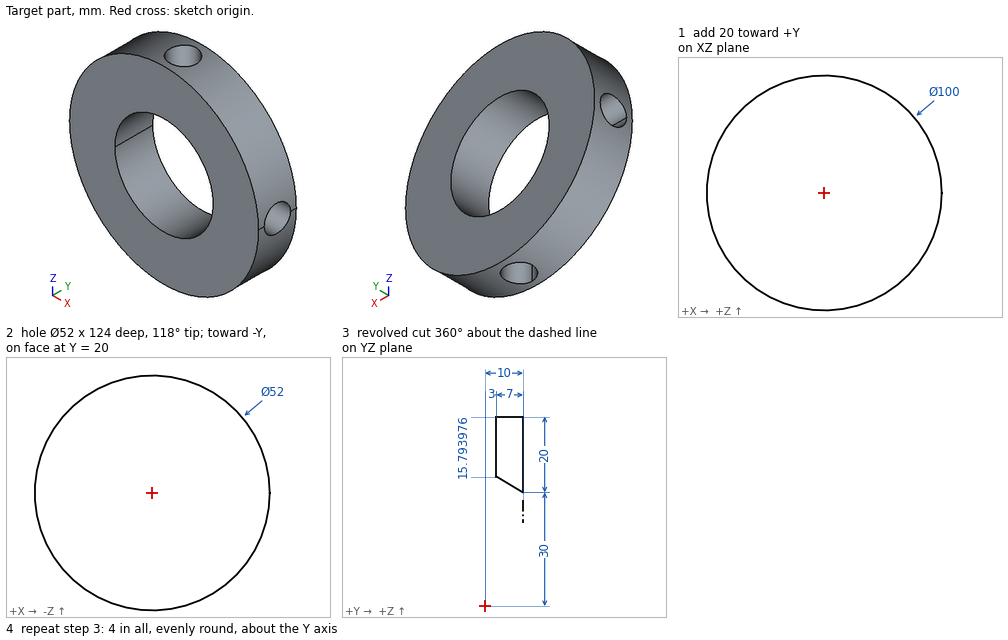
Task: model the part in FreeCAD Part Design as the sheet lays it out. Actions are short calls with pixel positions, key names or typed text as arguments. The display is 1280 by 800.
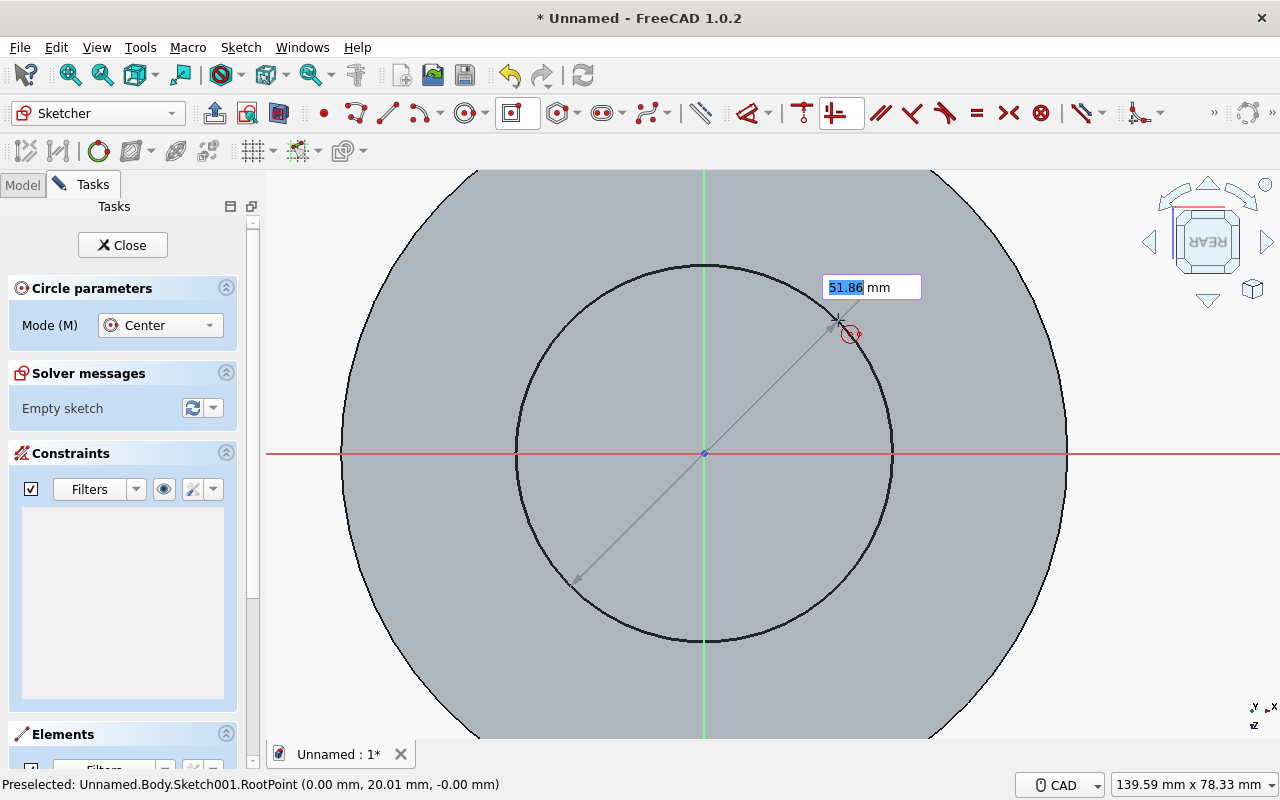
text(52)
key(Return)
key(Escape)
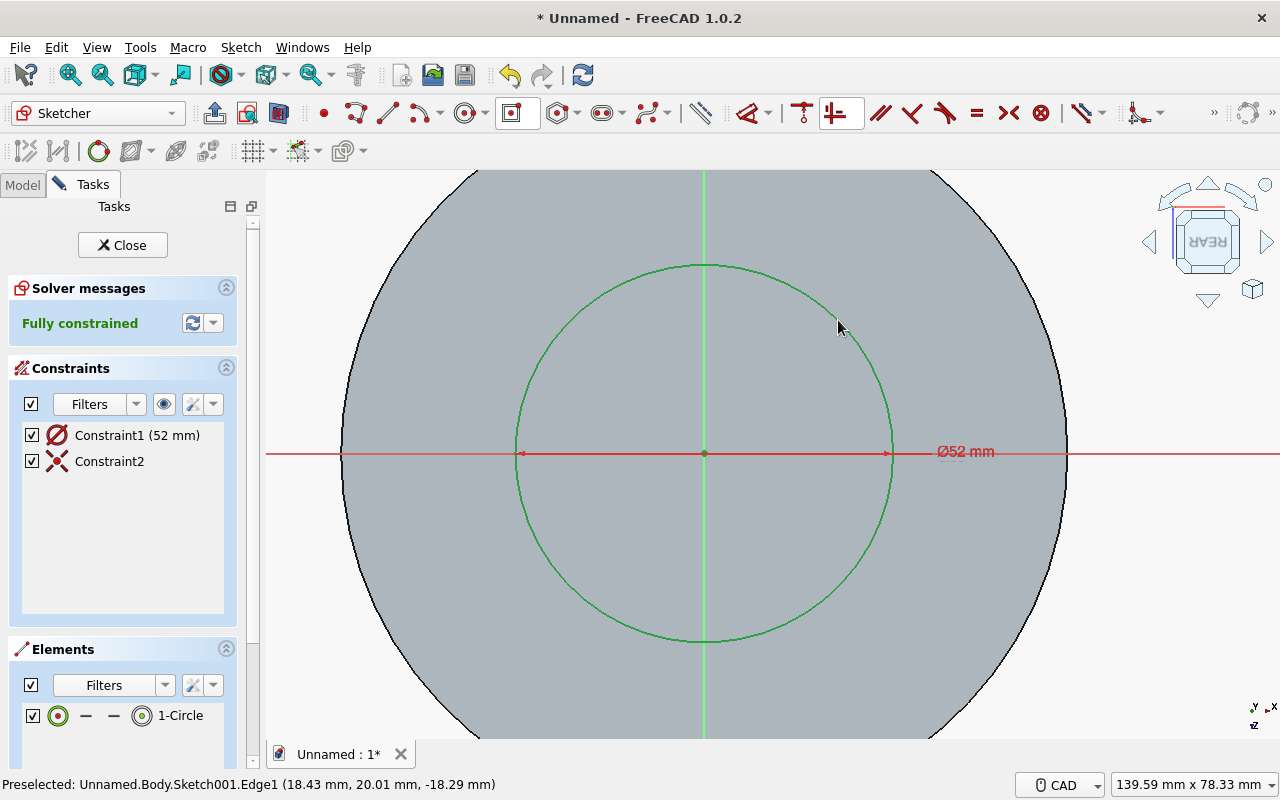
click(123, 245)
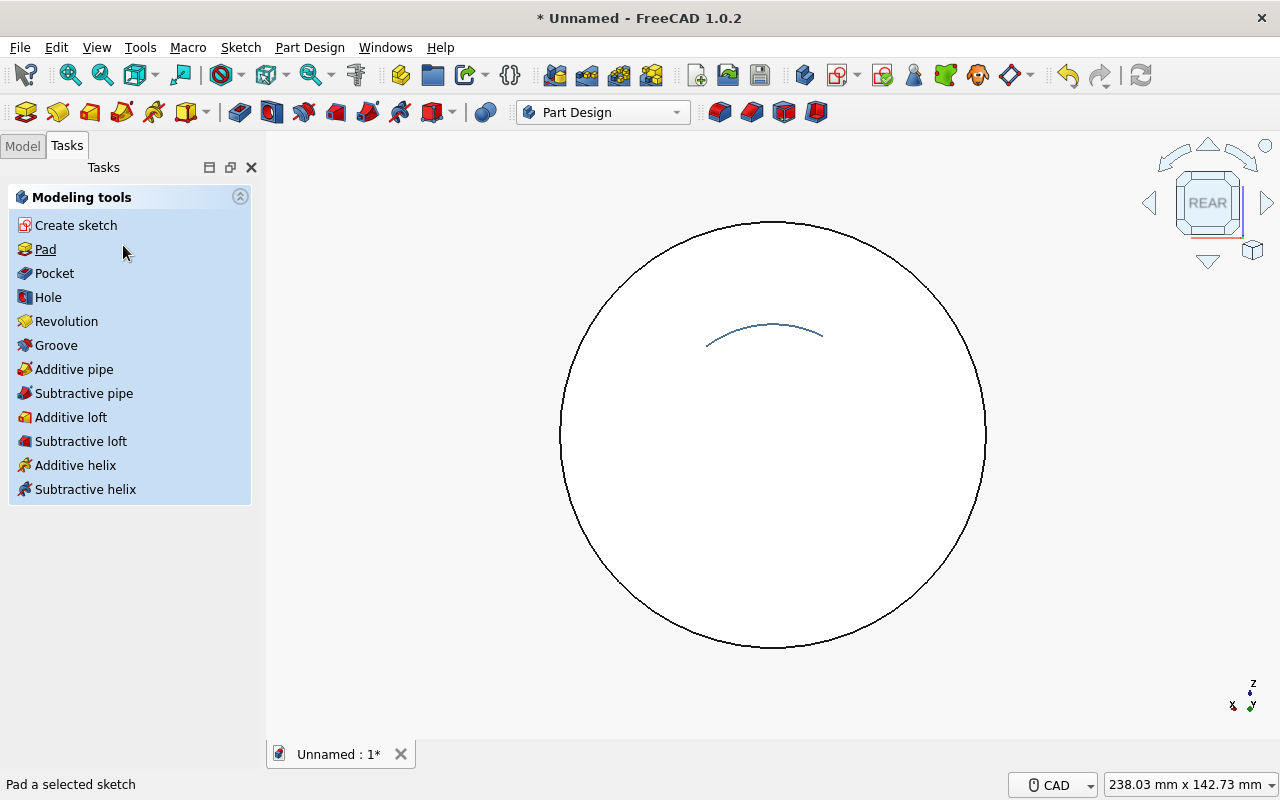
click(272, 112)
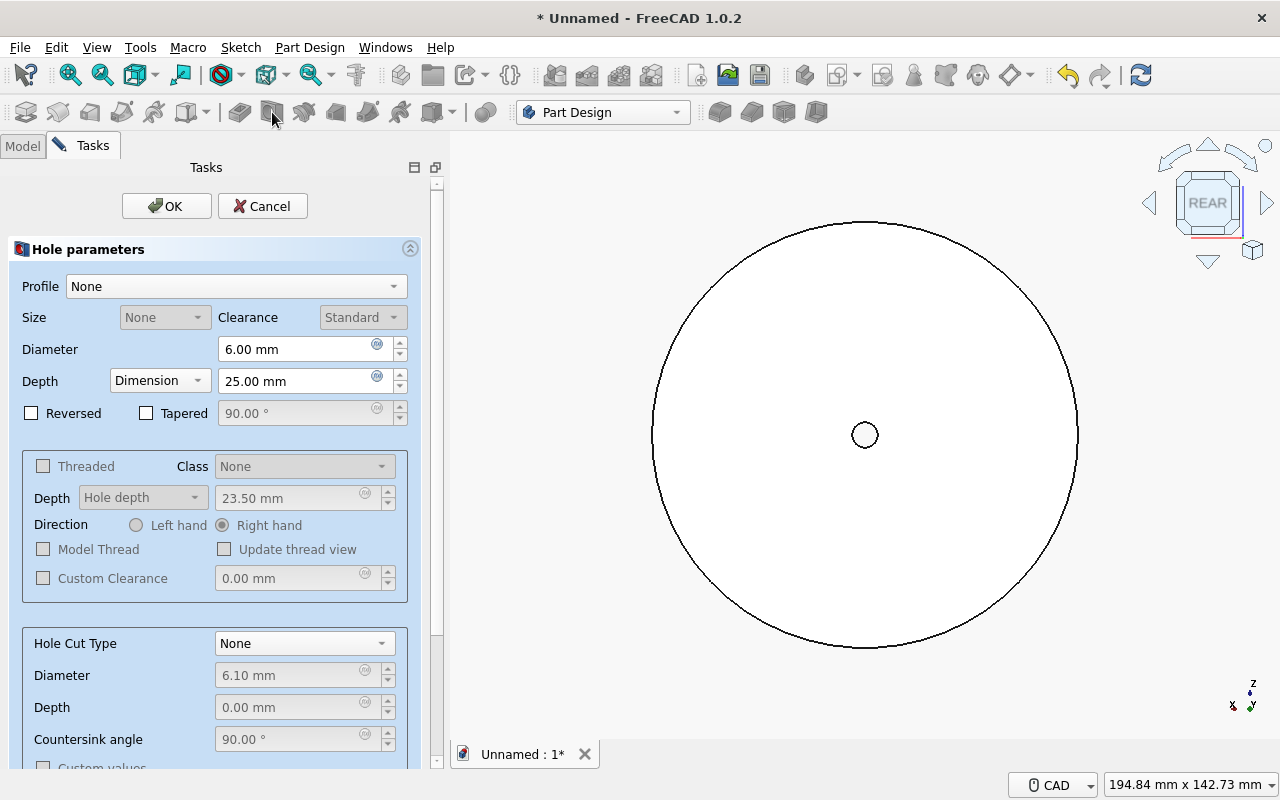
triple_click(305, 349)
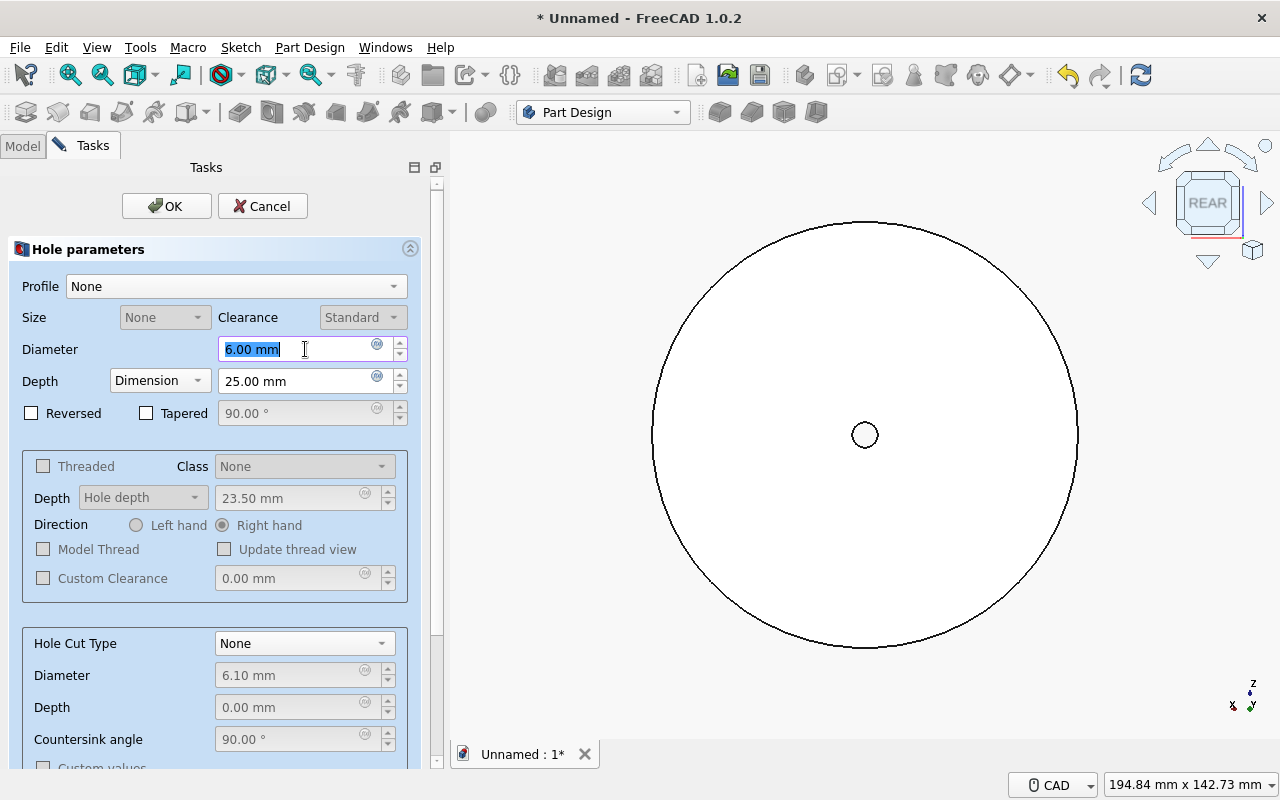
text(52)
key(Tab)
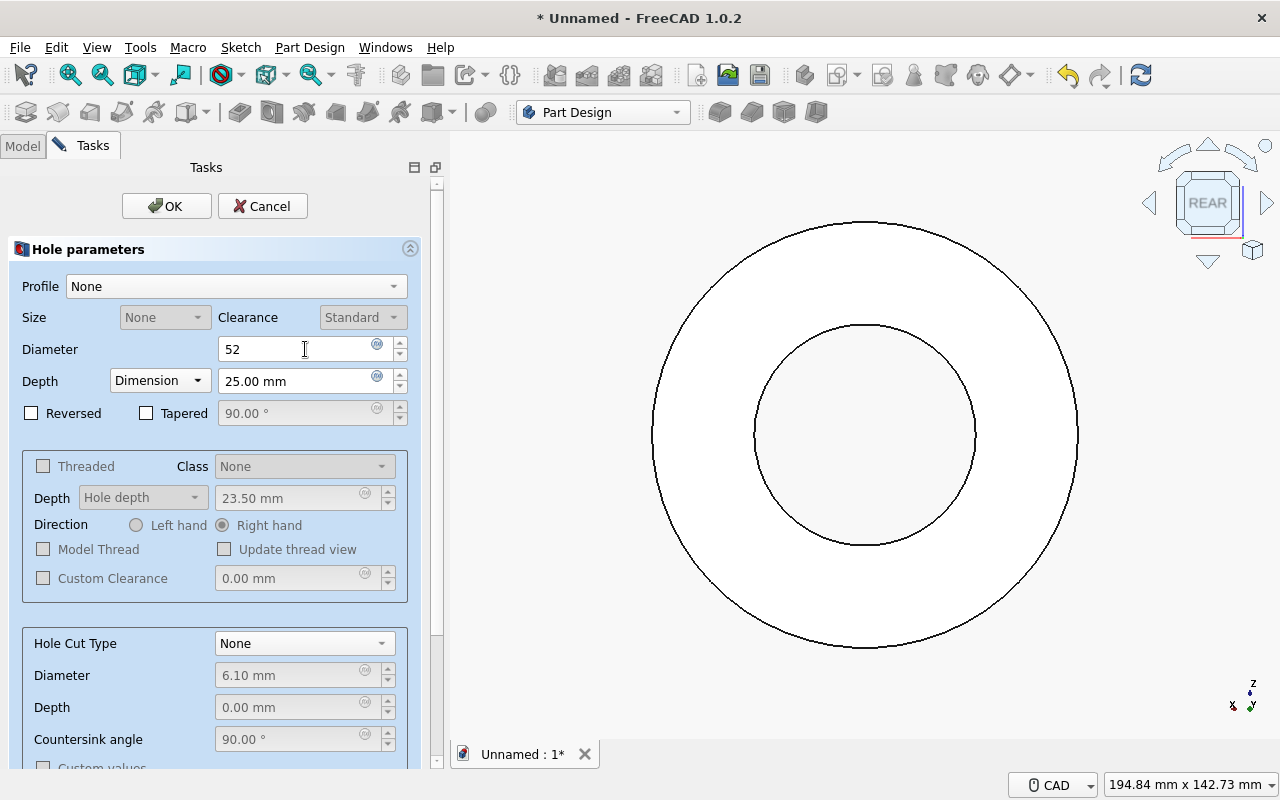
triple_click(305, 381)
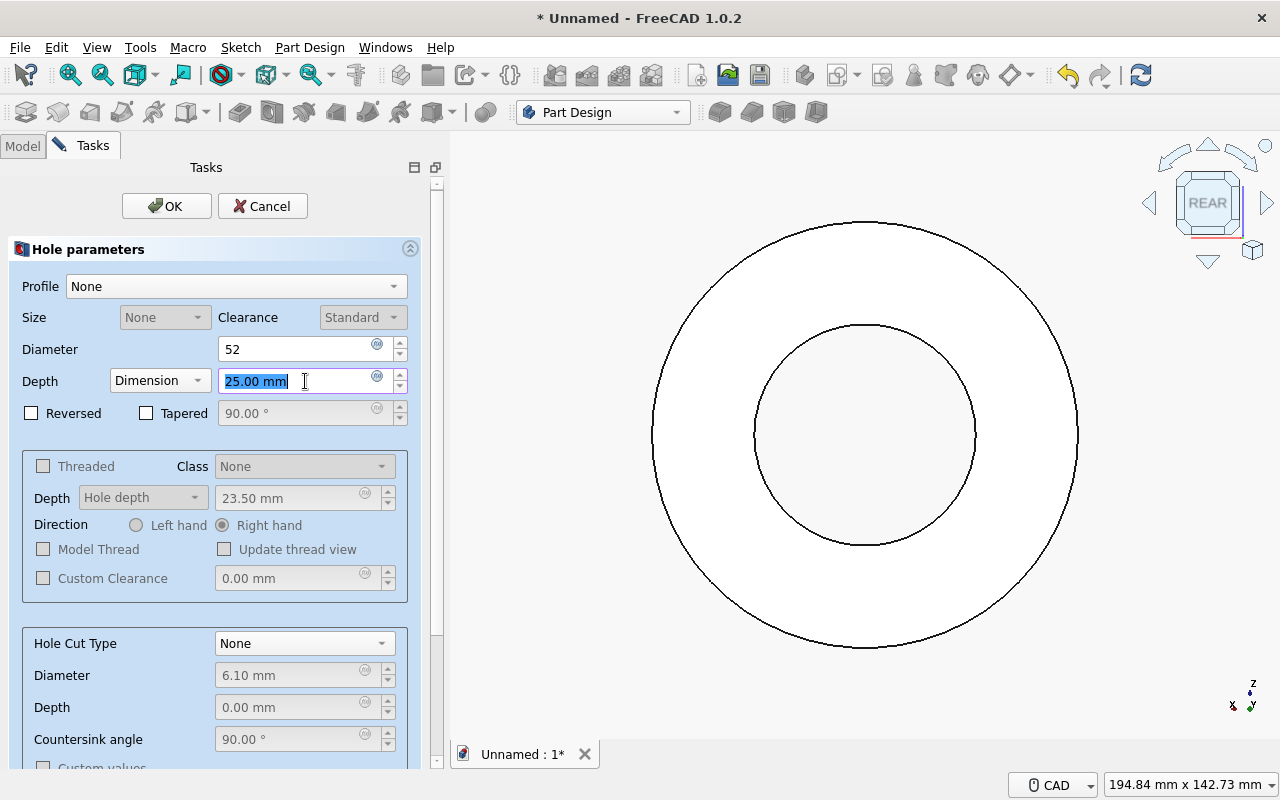
text(124)
key(Tab)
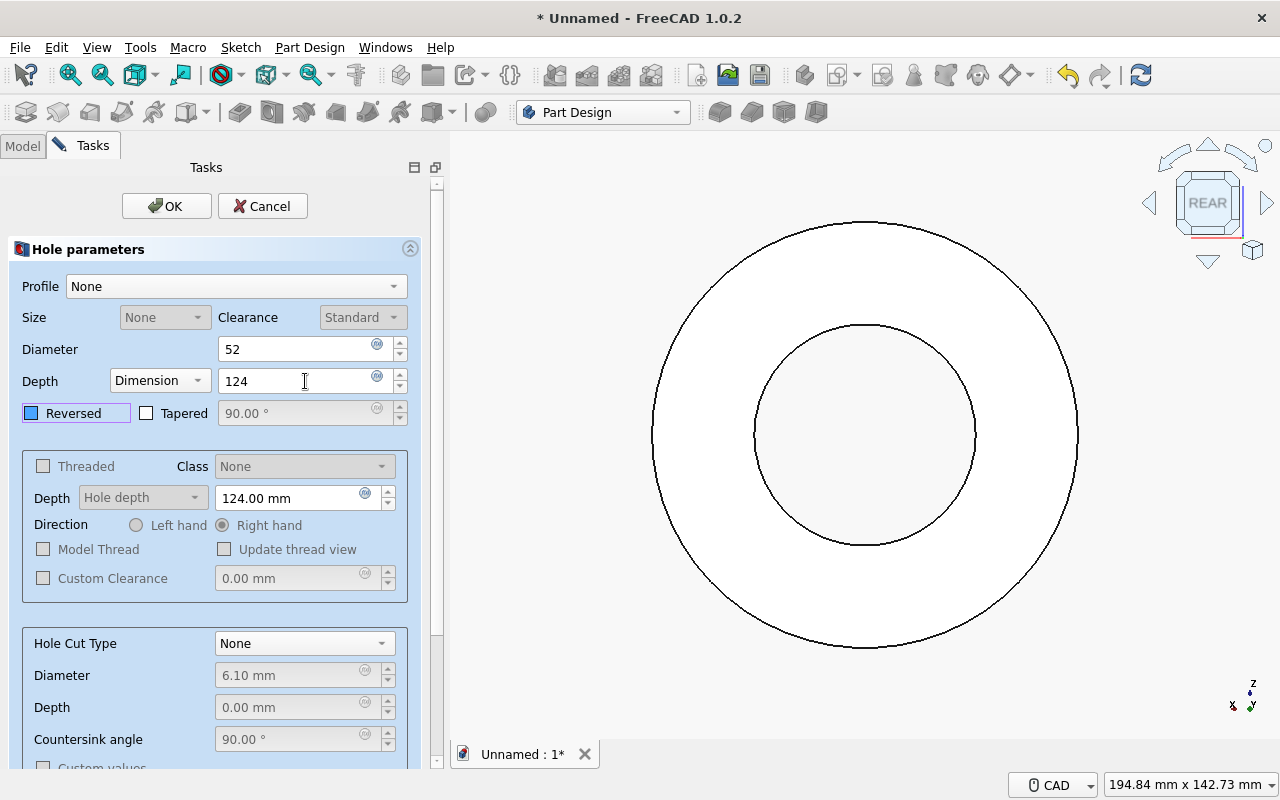
click(167, 206)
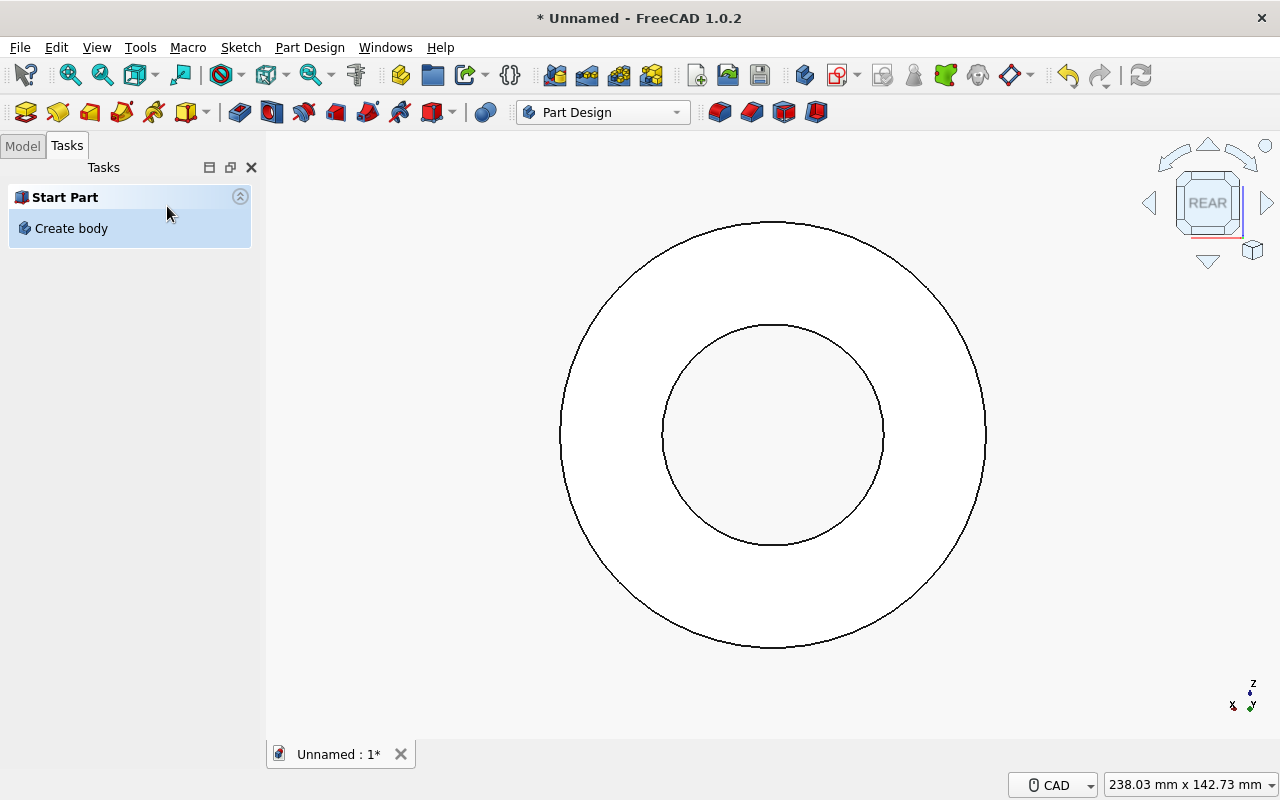
click(838, 76)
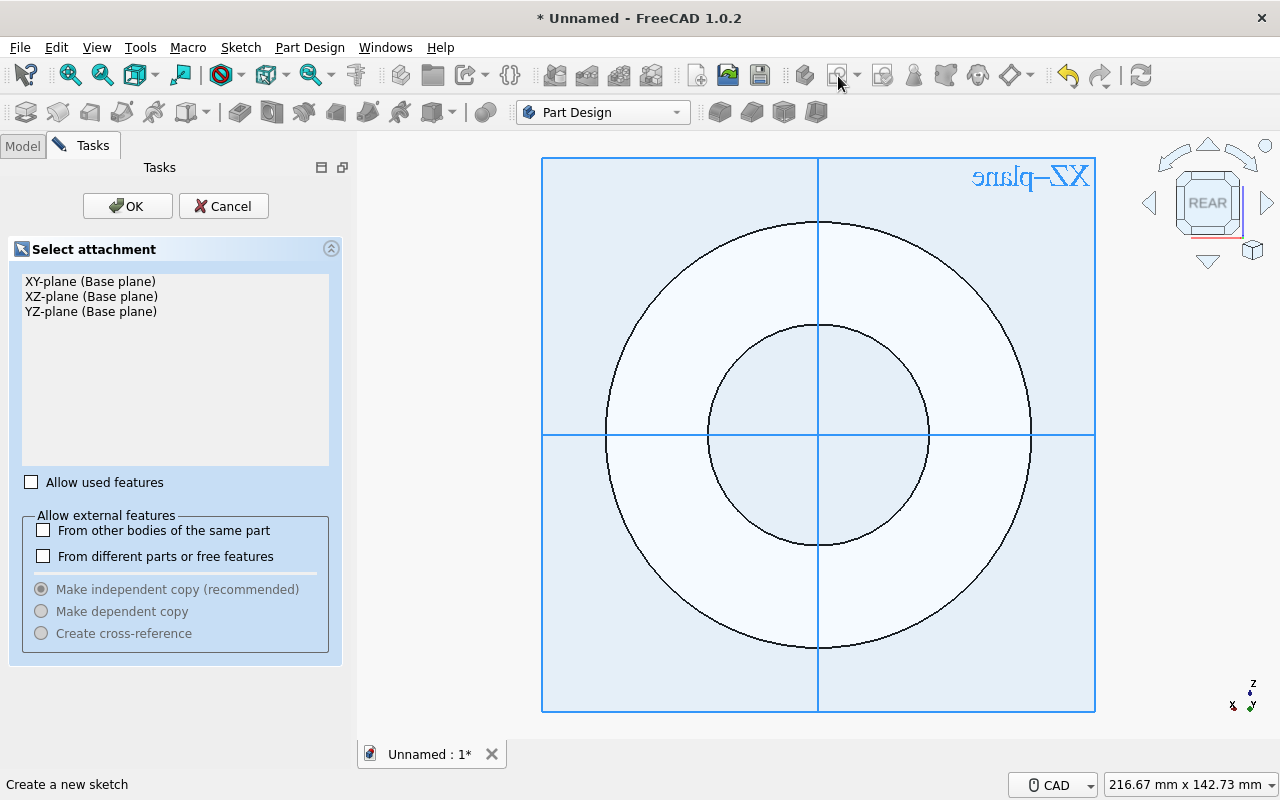
click(82, 312)